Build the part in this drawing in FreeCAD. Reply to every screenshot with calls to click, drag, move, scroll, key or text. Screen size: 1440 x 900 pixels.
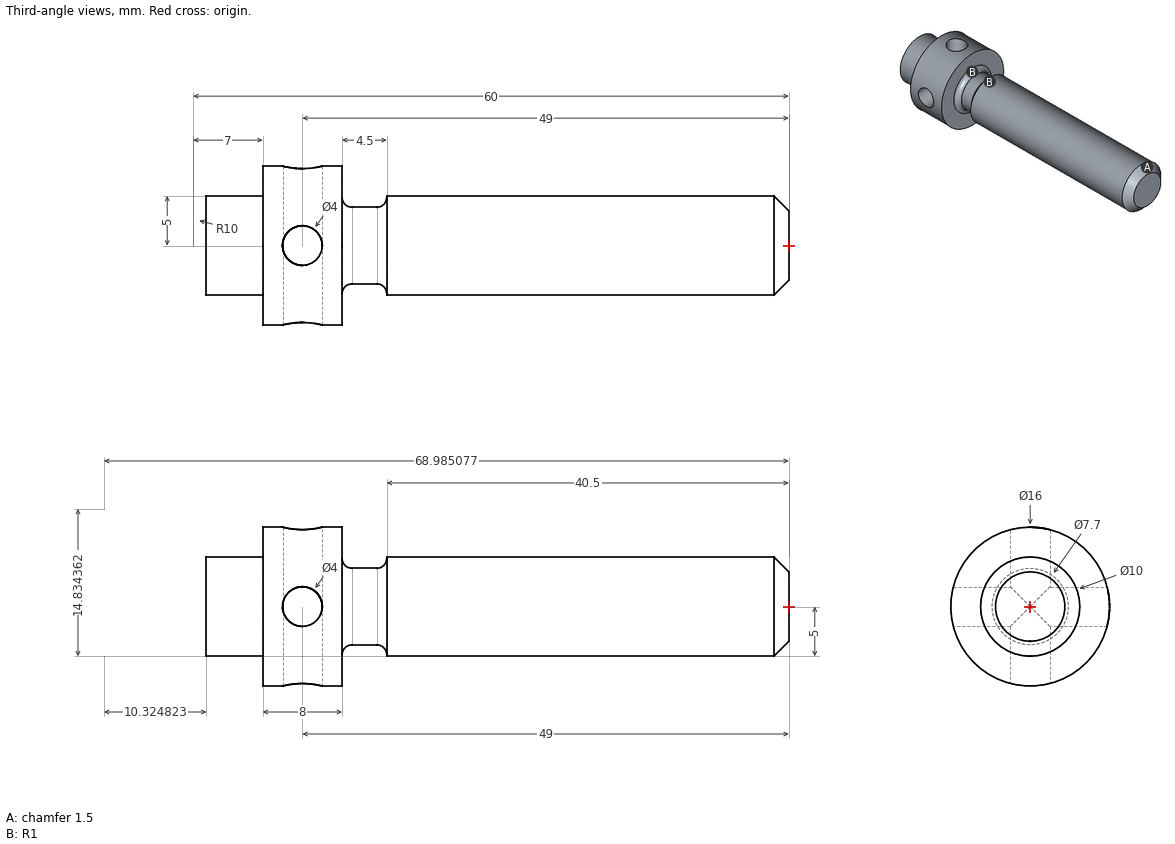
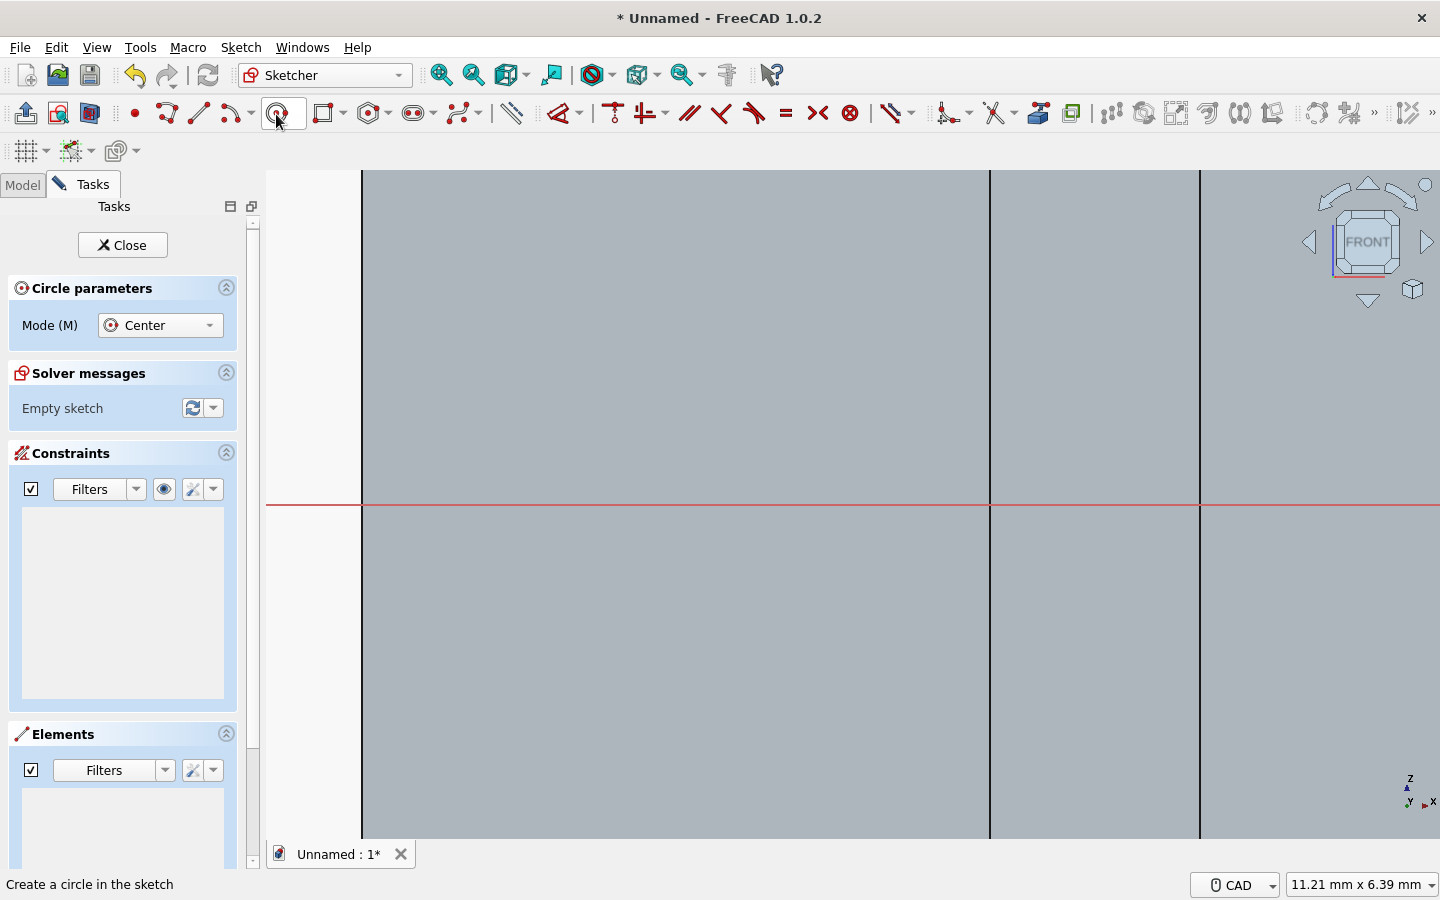
click(781, 504)
click(929, 356)
key(Escape)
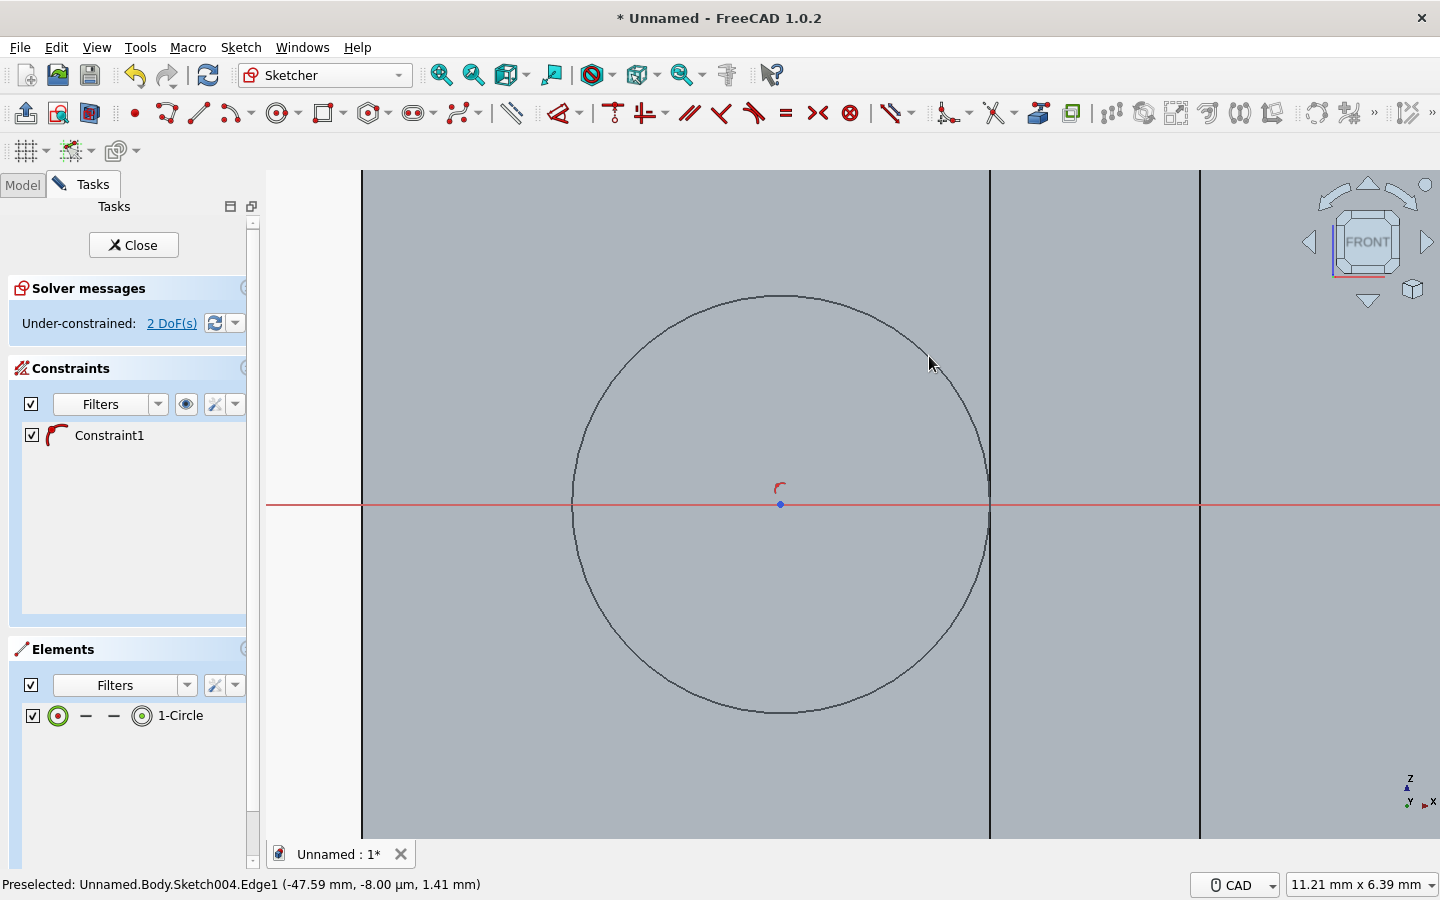
key(d)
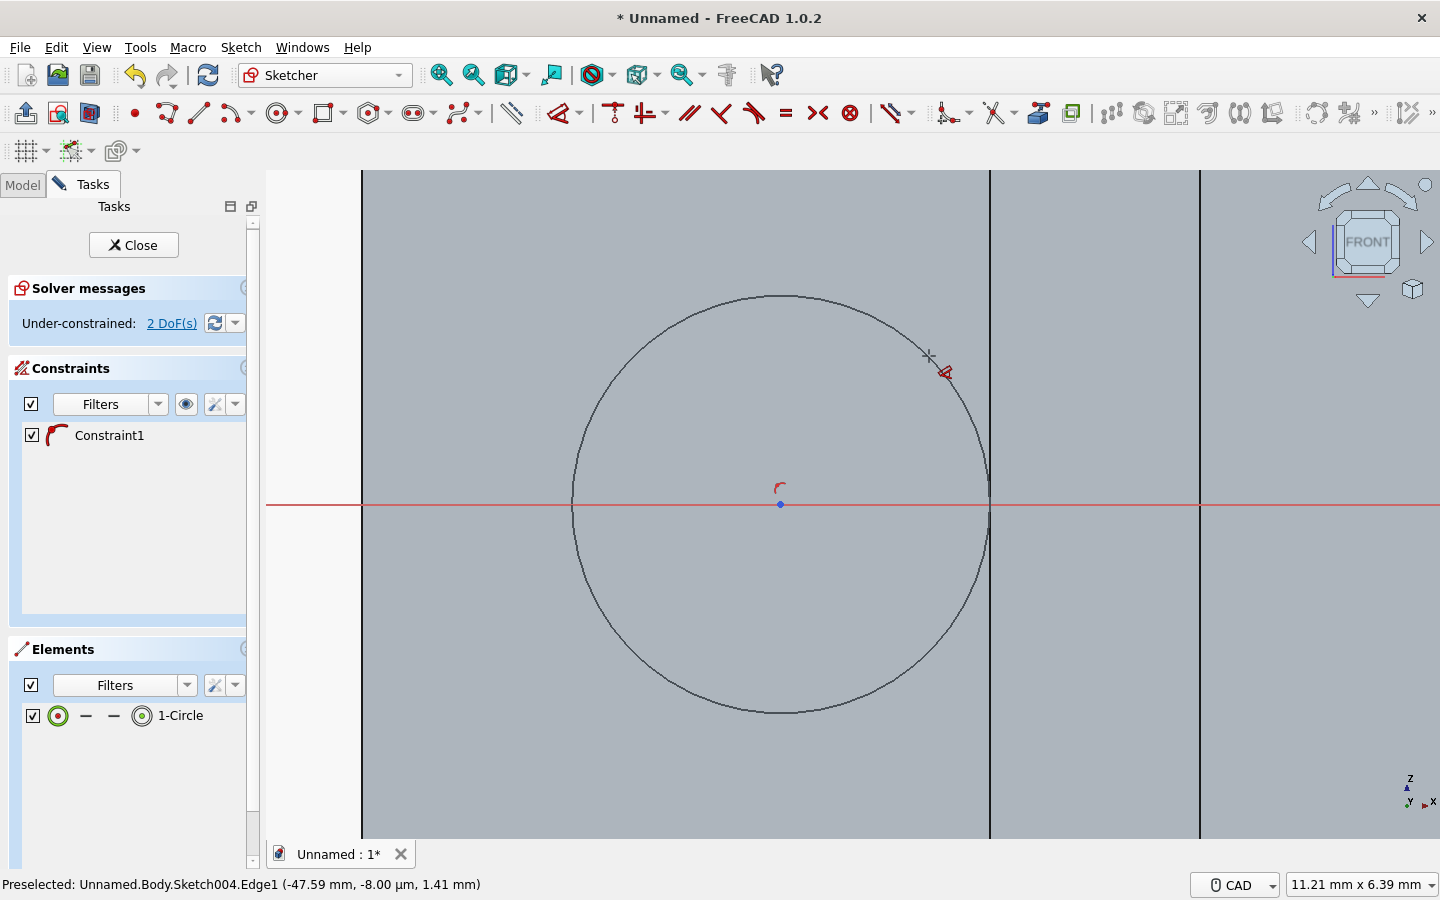
click(928, 356)
click(951, 333)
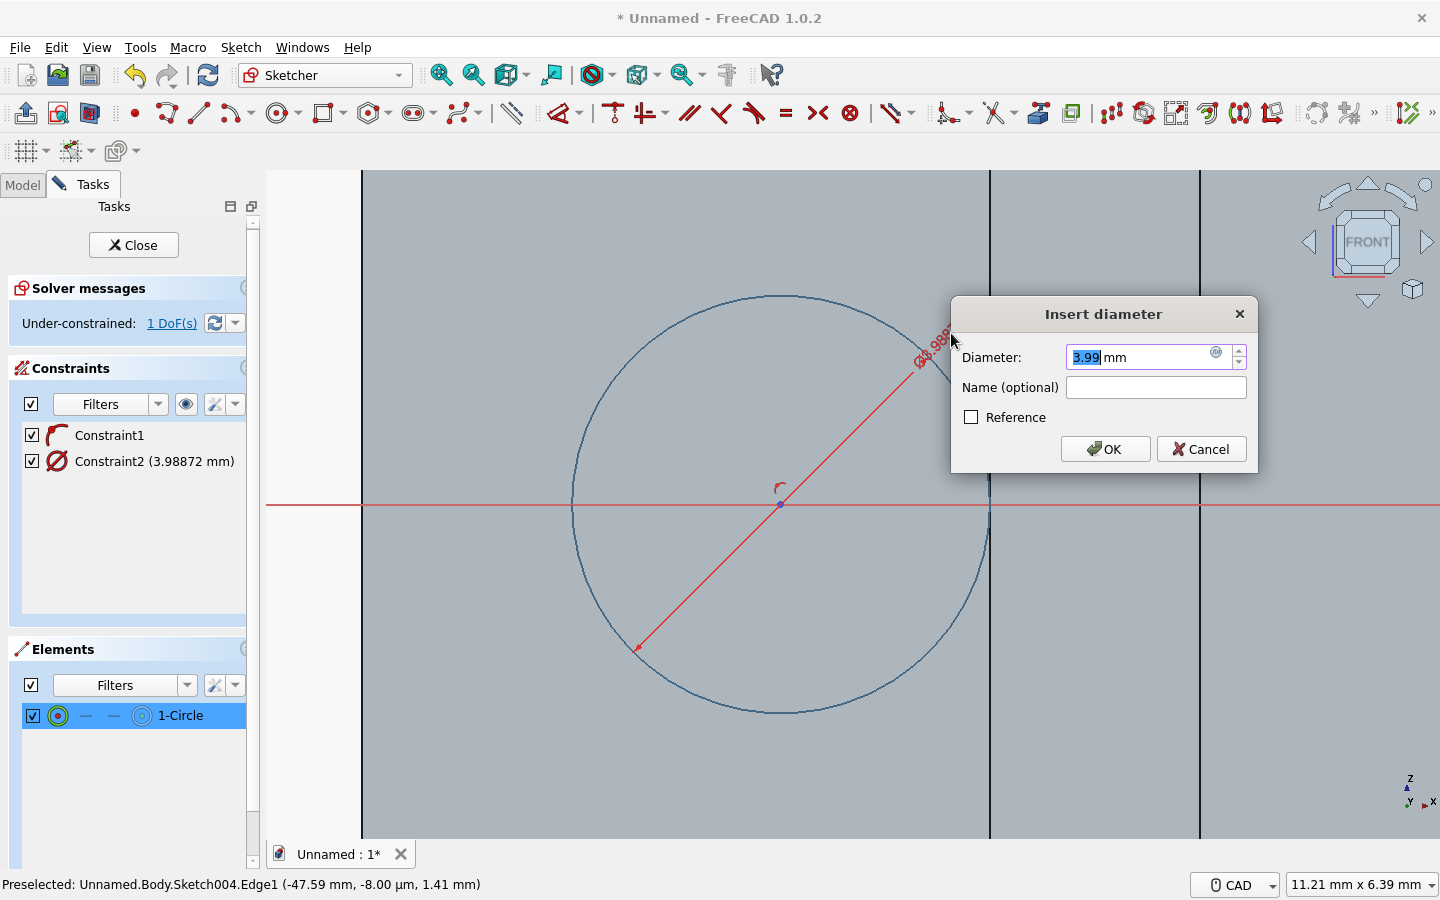
text(4)
key(Return)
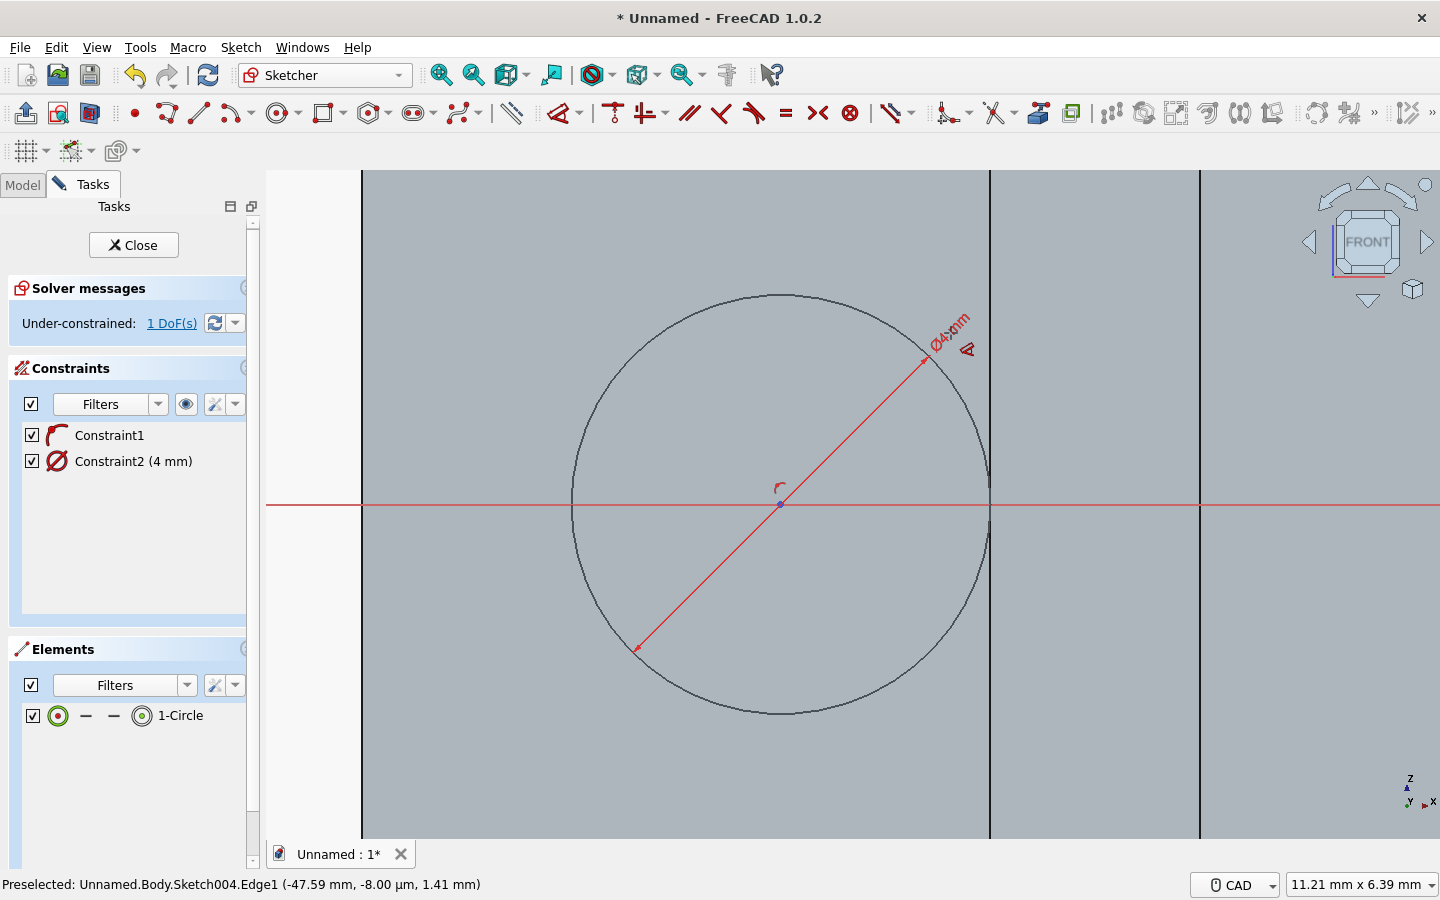
click(781, 504)
click(1028, 538)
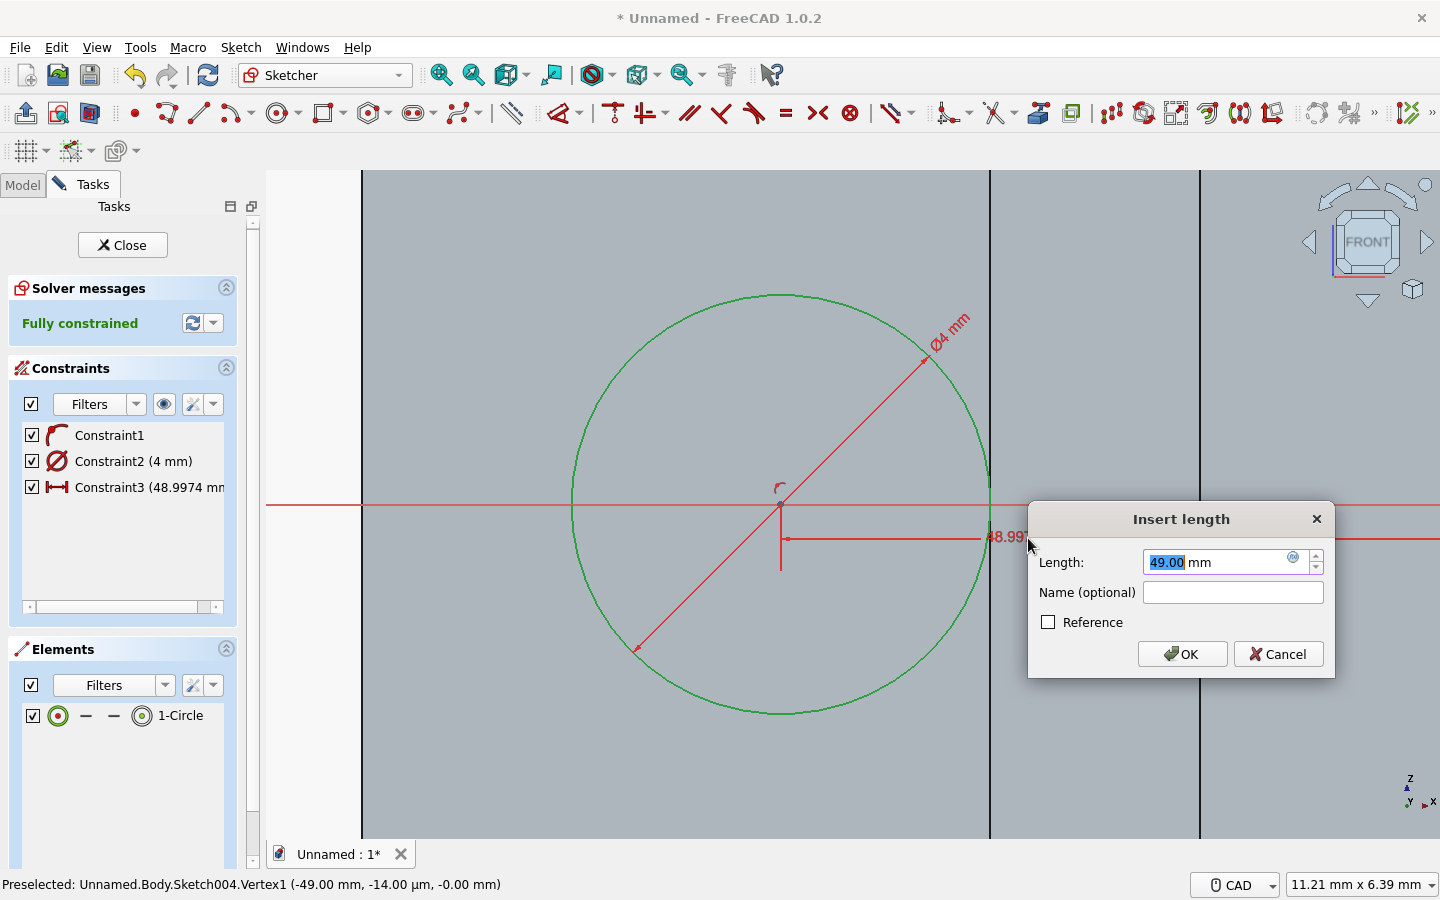
text(49)
key(Return)
key(Escape)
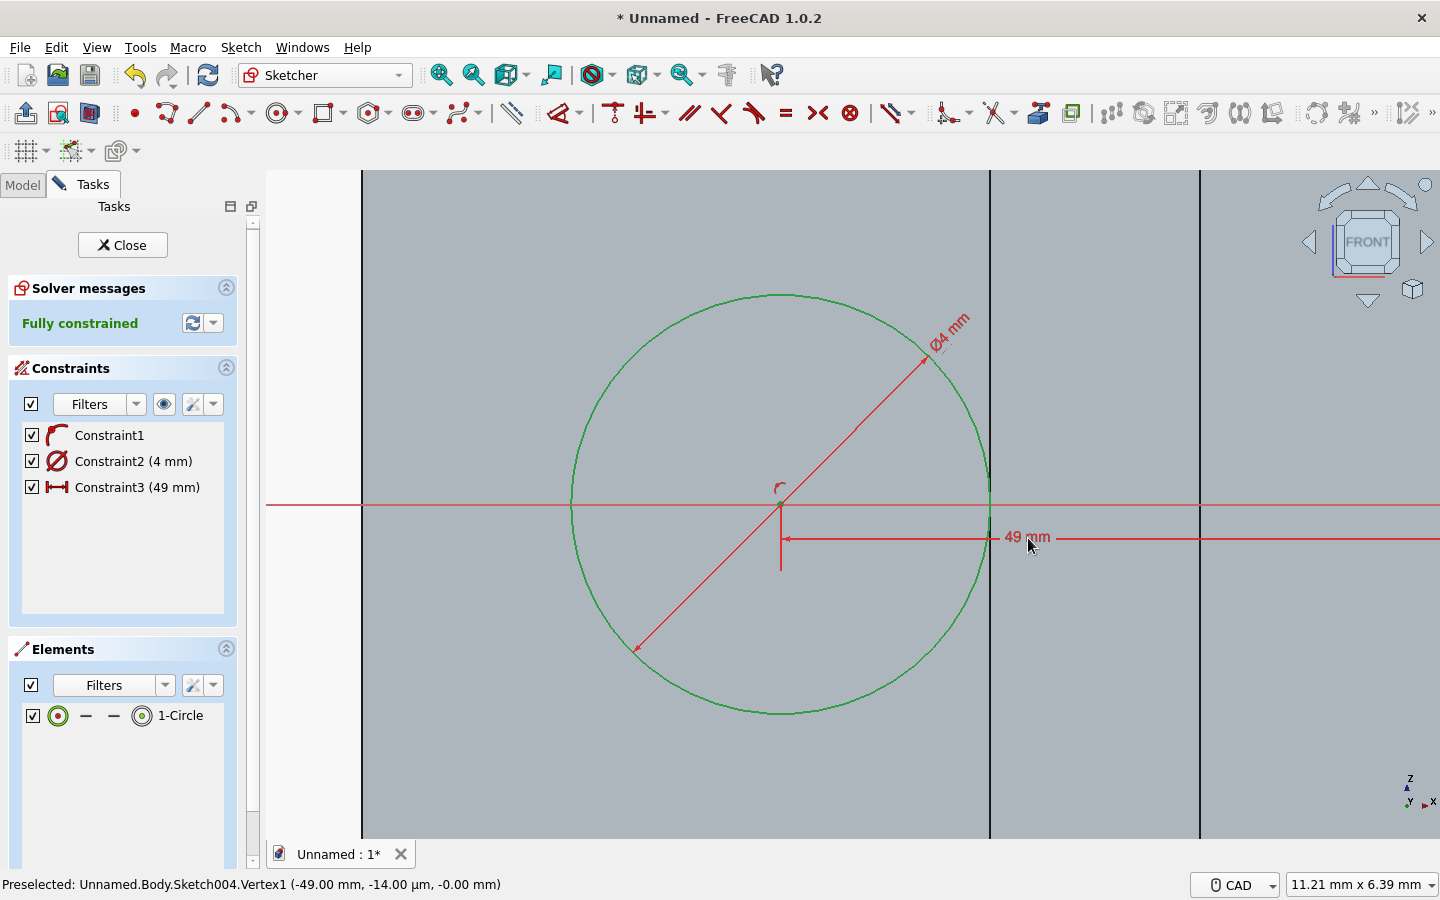
click(123, 245)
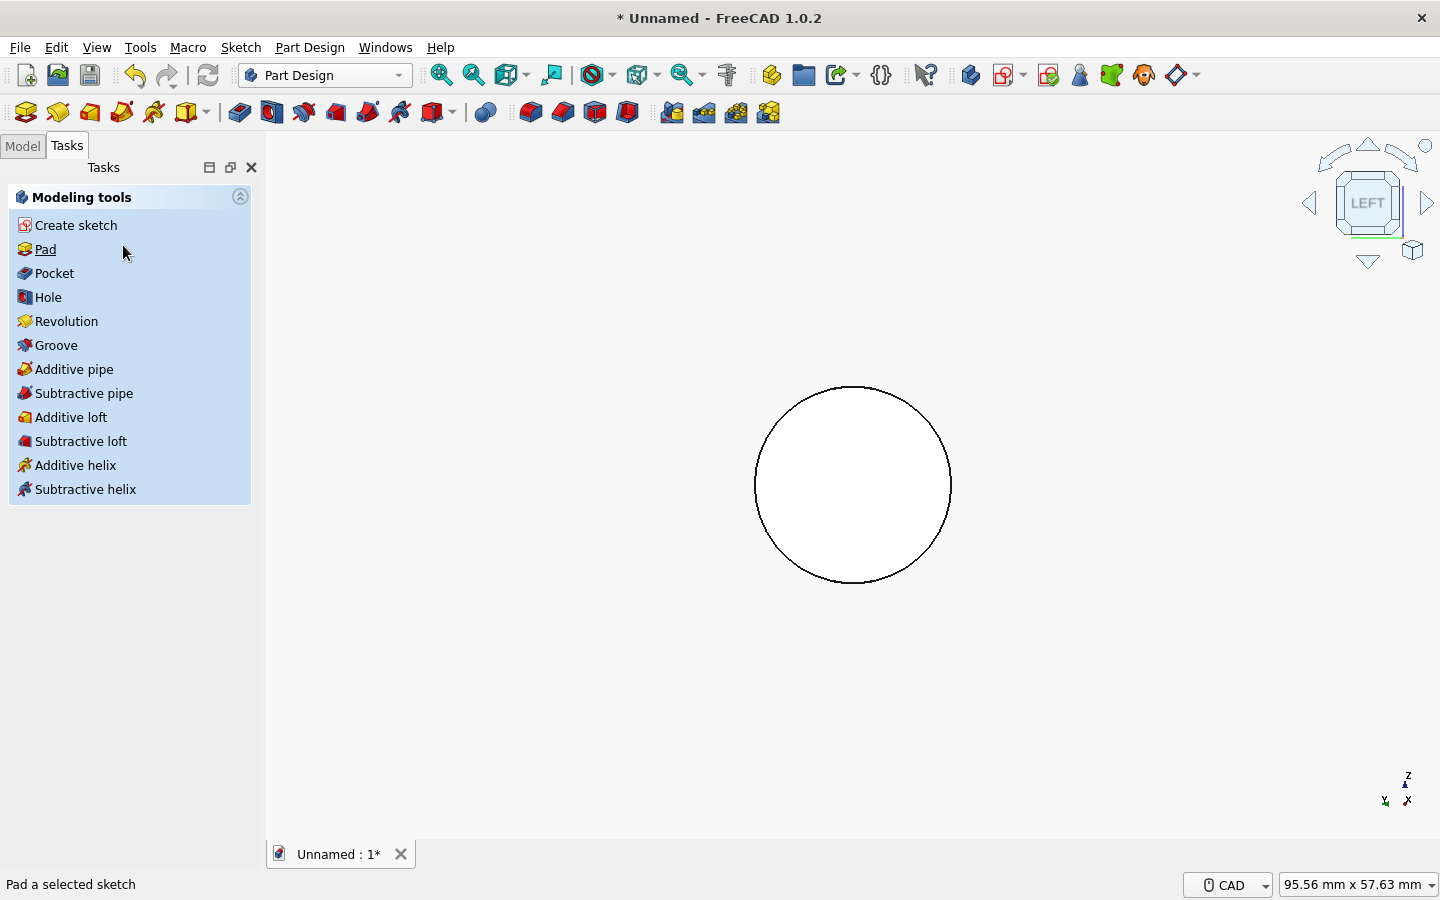
click(240, 112)